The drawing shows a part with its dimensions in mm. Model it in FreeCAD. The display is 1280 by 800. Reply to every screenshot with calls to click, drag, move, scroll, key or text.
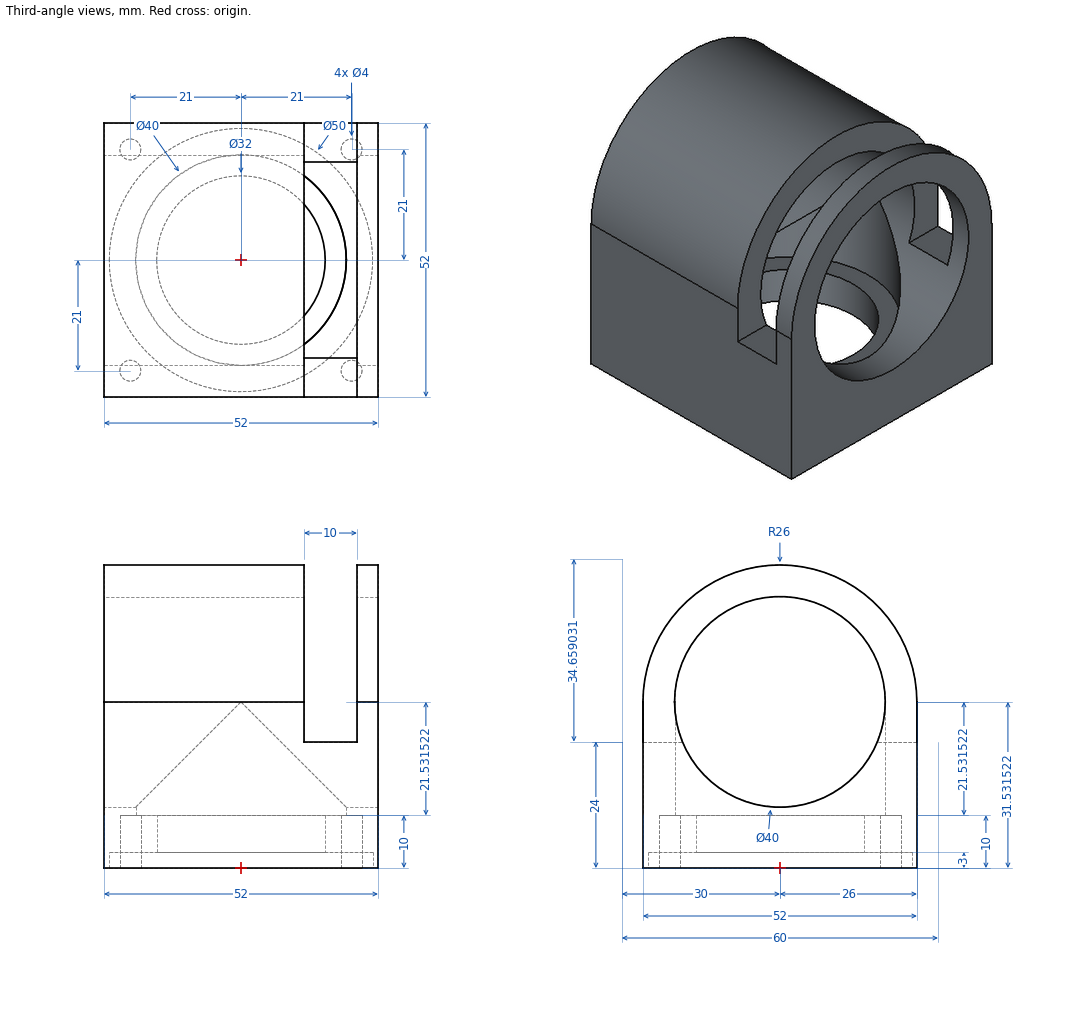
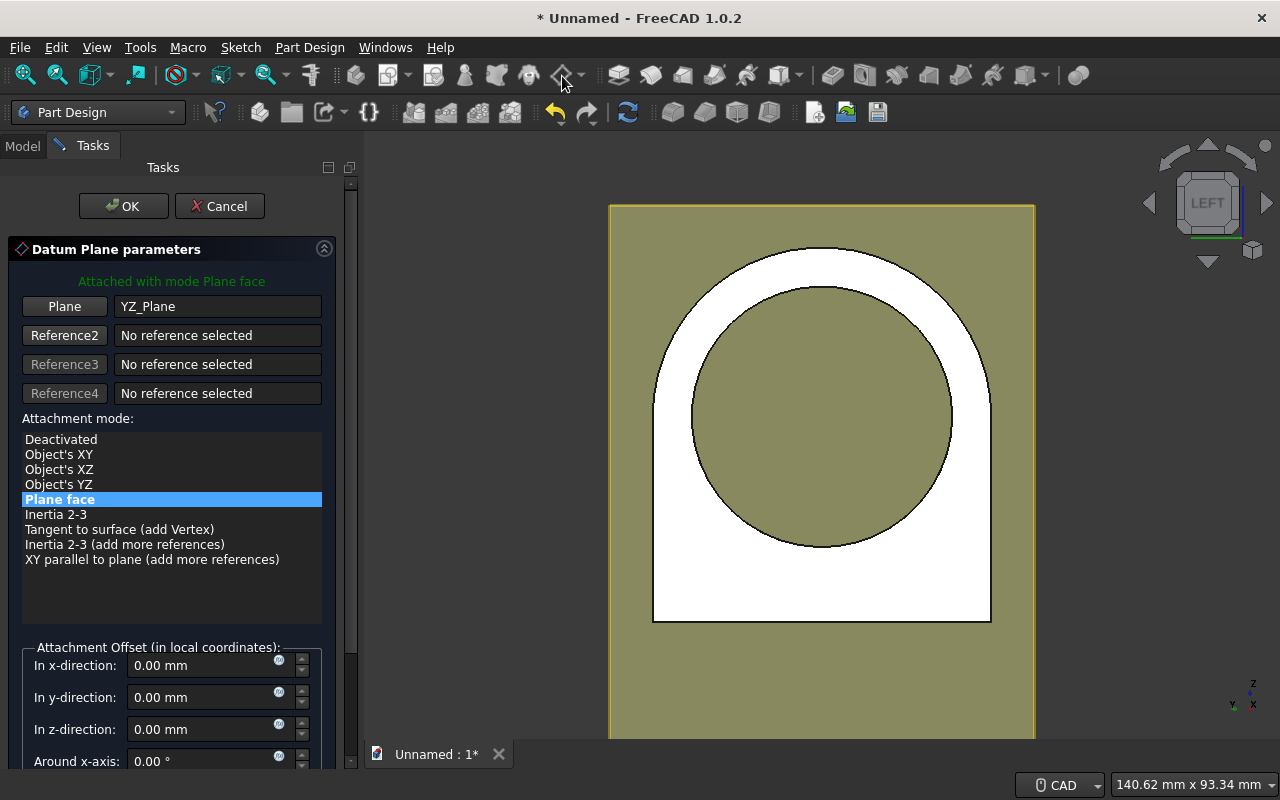
triple_click(210, 729)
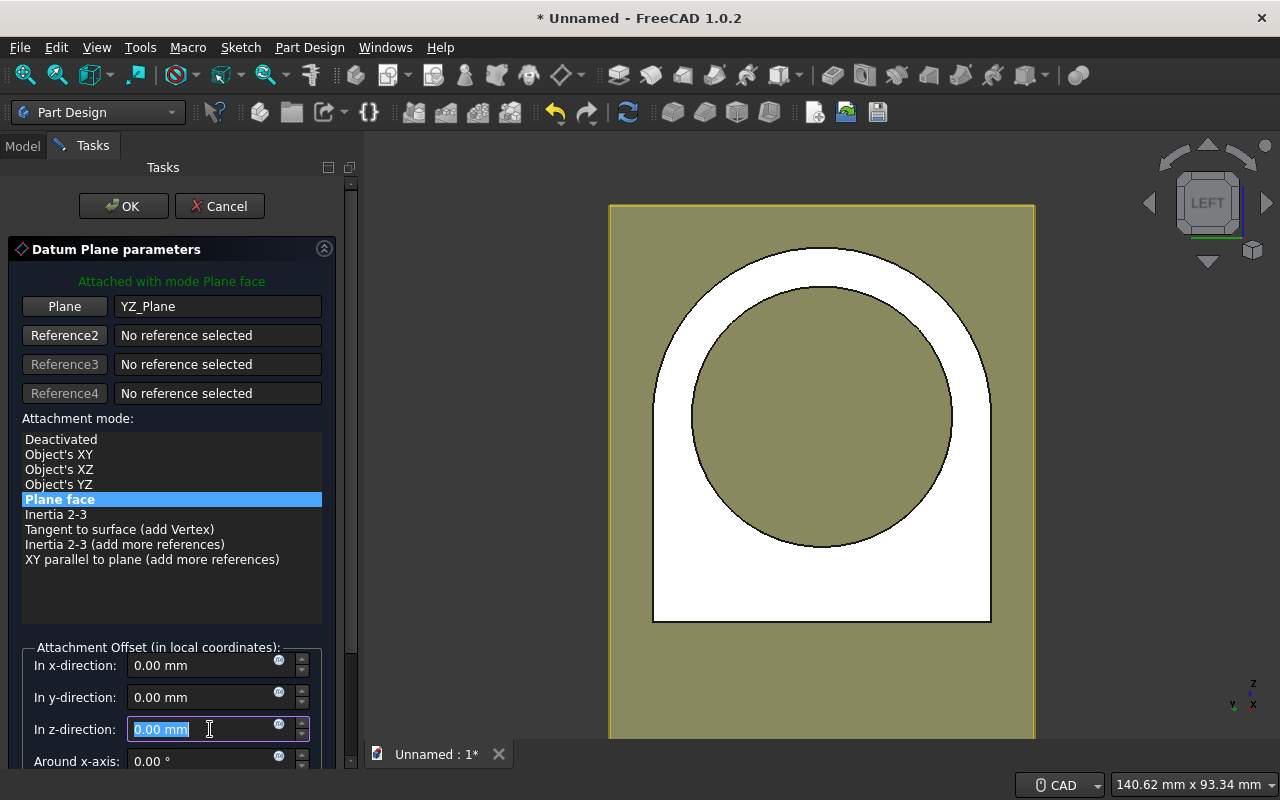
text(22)
key(Tab)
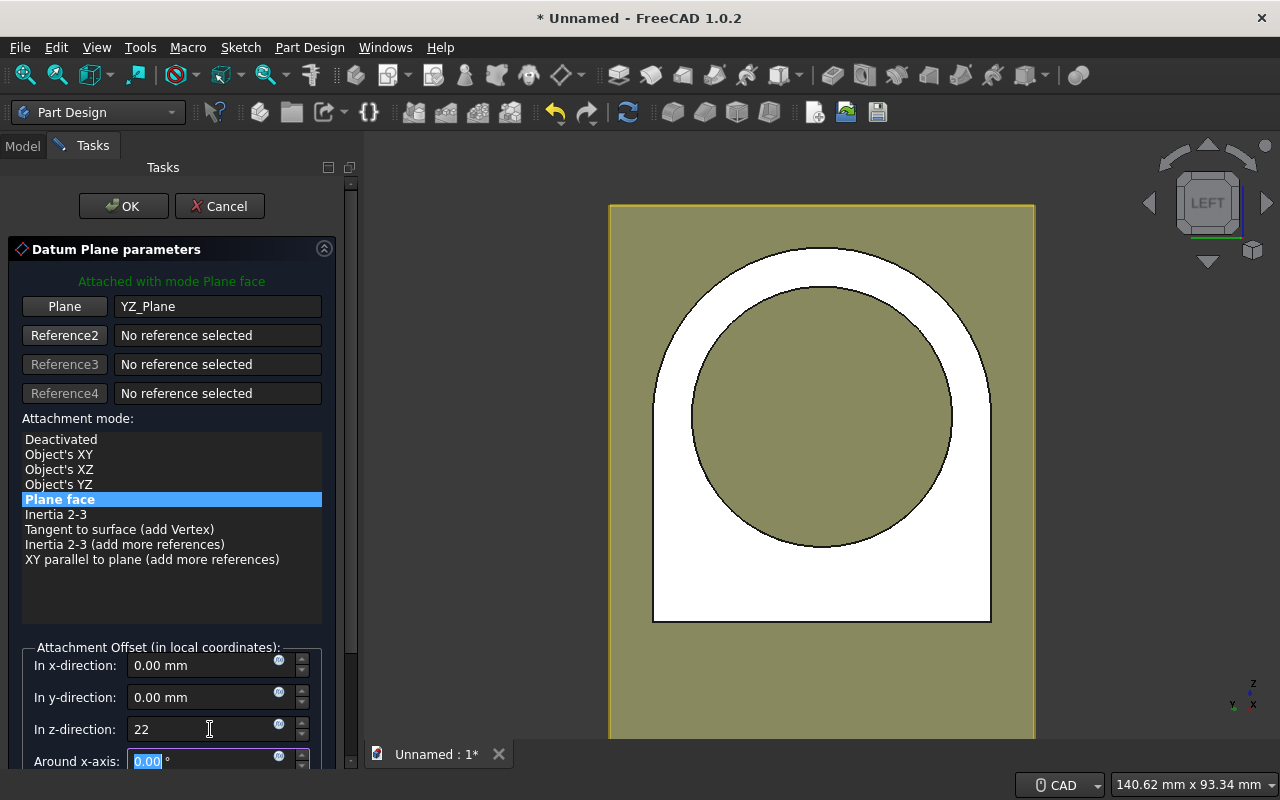
click(124, 206)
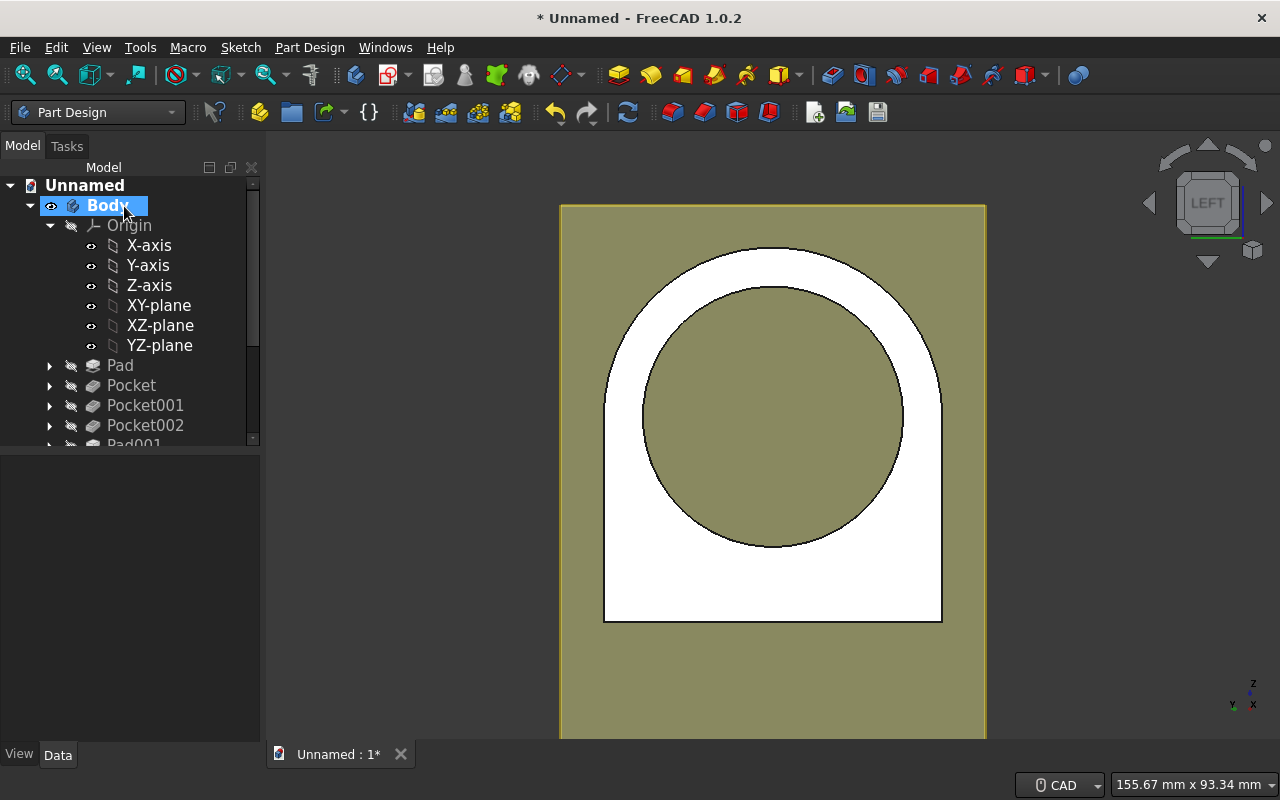
scroll(100, 321, down, 3)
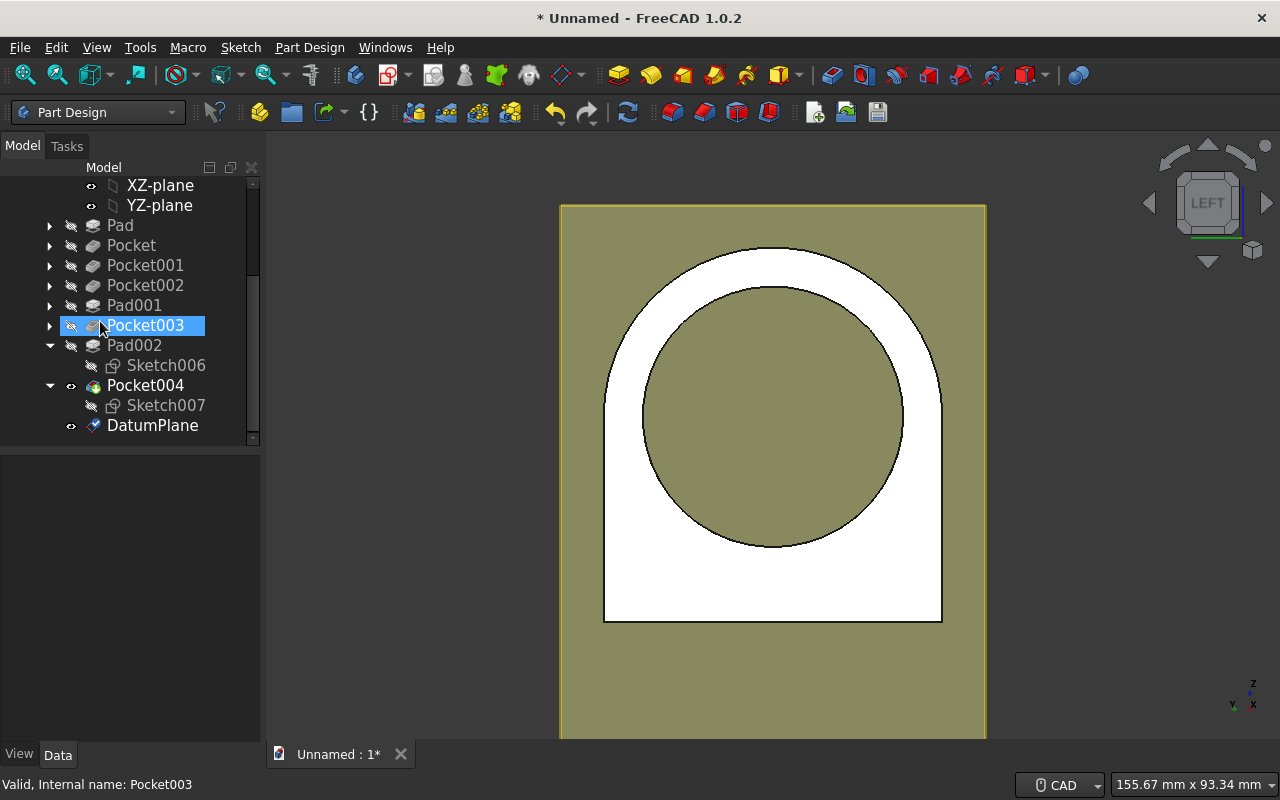
click(116, 426)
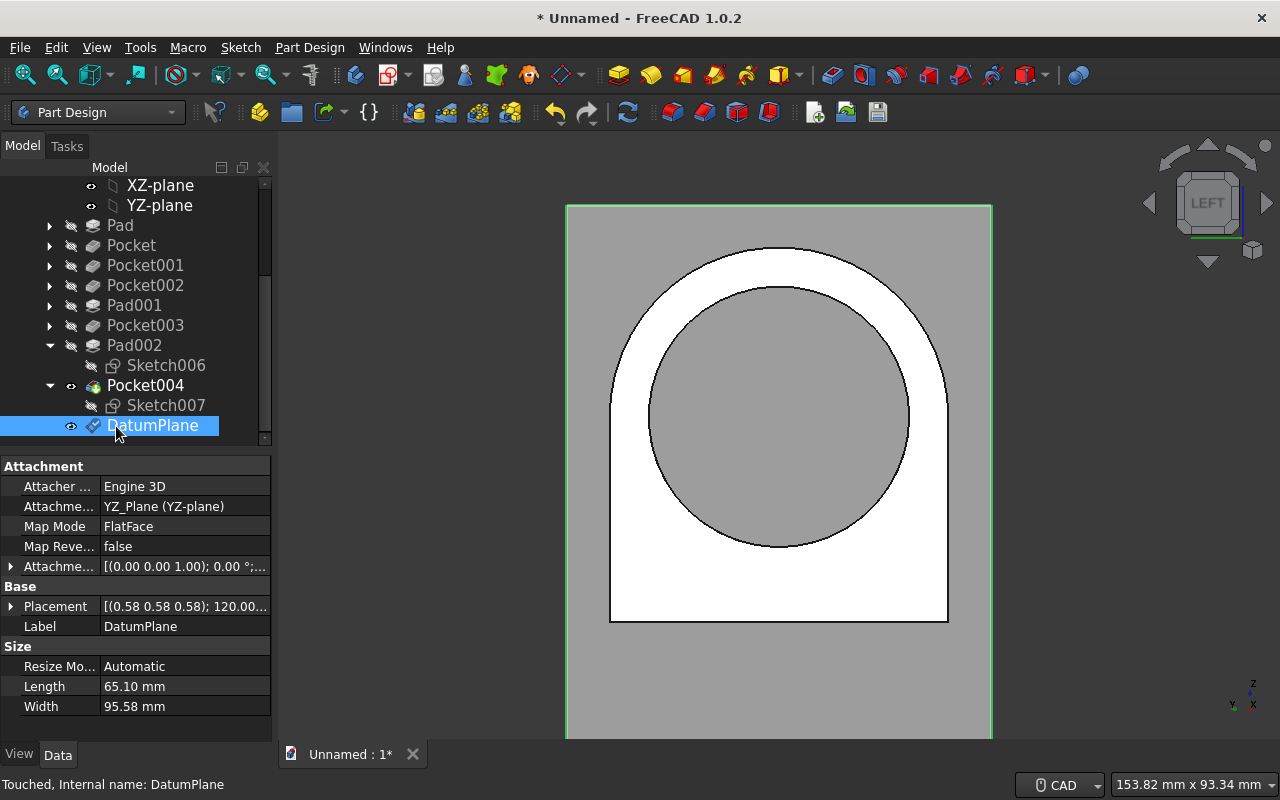
click(388, 76)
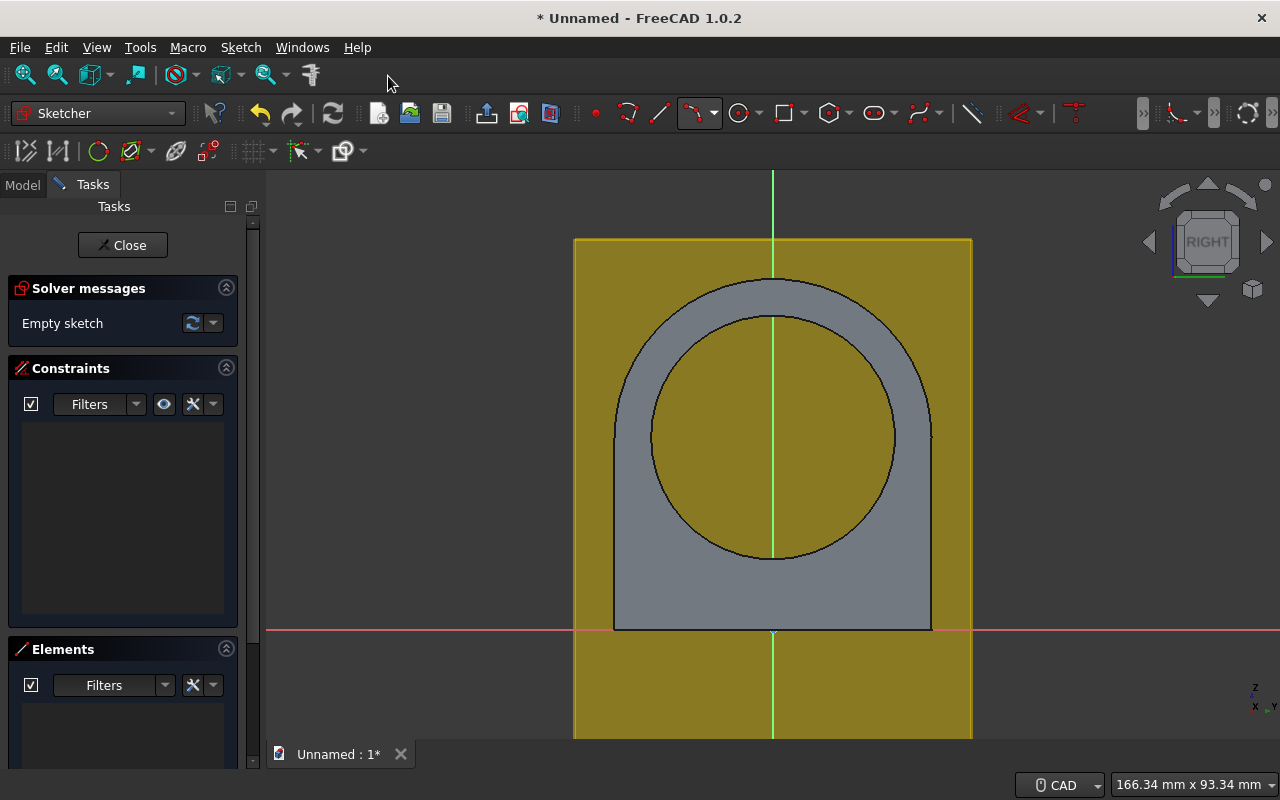
click(552, 114)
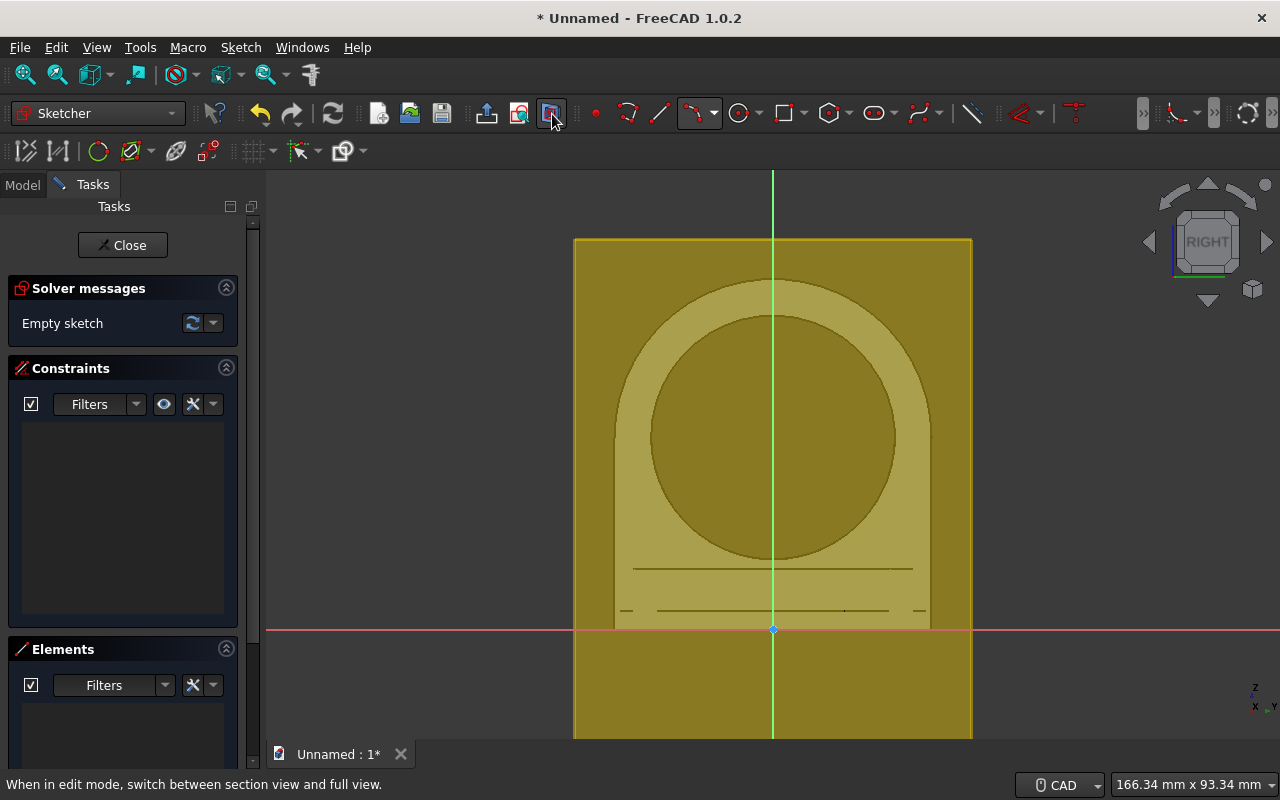
click(784, 114)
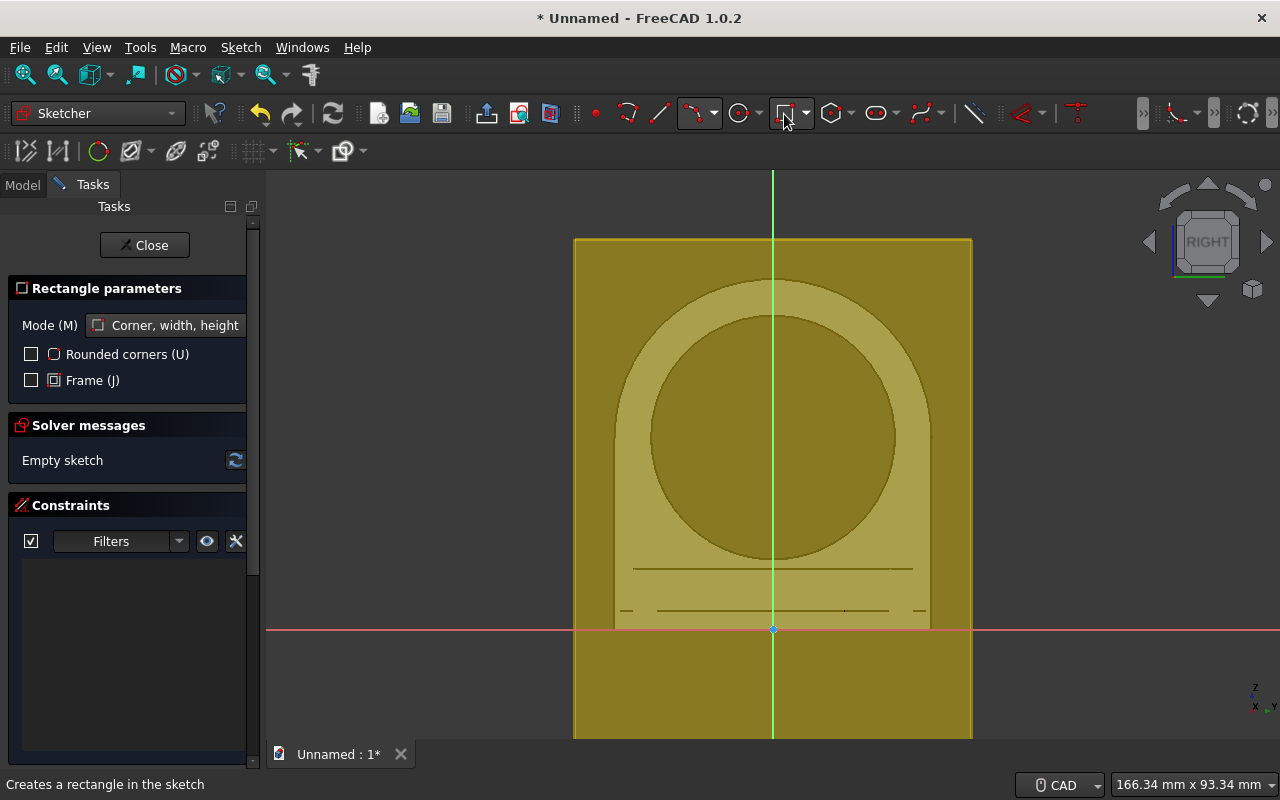
click(590, 272)
click(956, 483)
key(Escape)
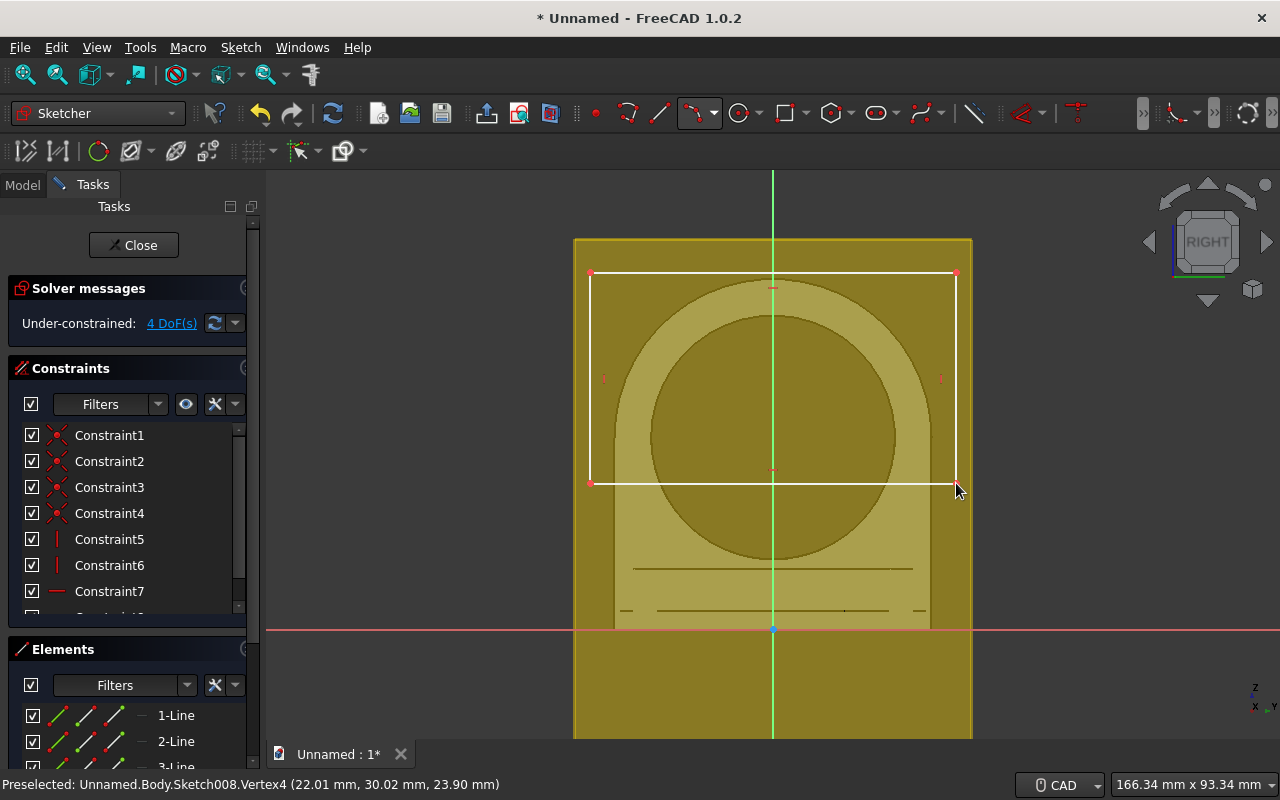
click(1022, 114)